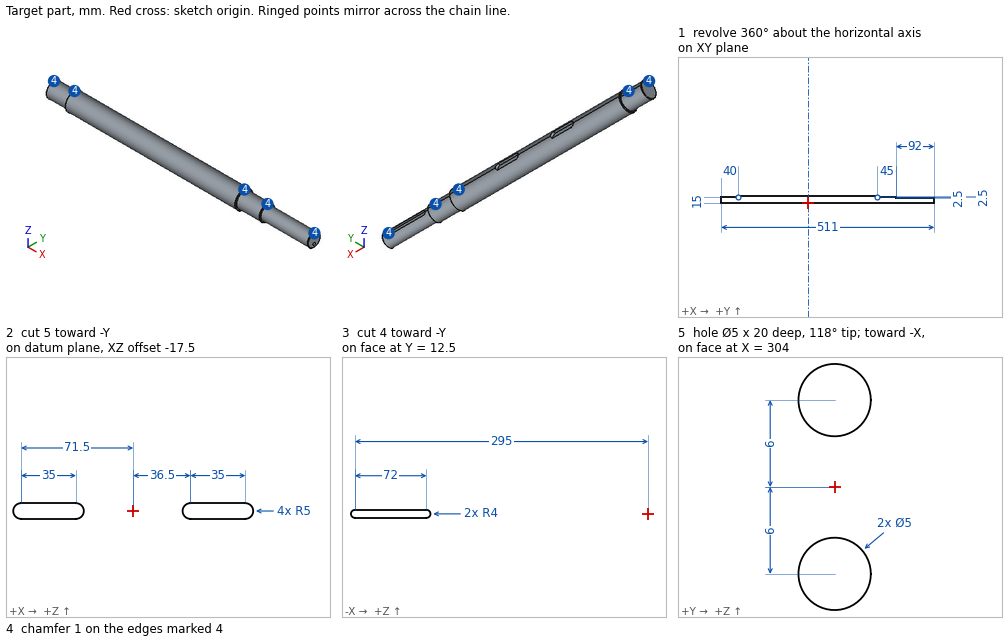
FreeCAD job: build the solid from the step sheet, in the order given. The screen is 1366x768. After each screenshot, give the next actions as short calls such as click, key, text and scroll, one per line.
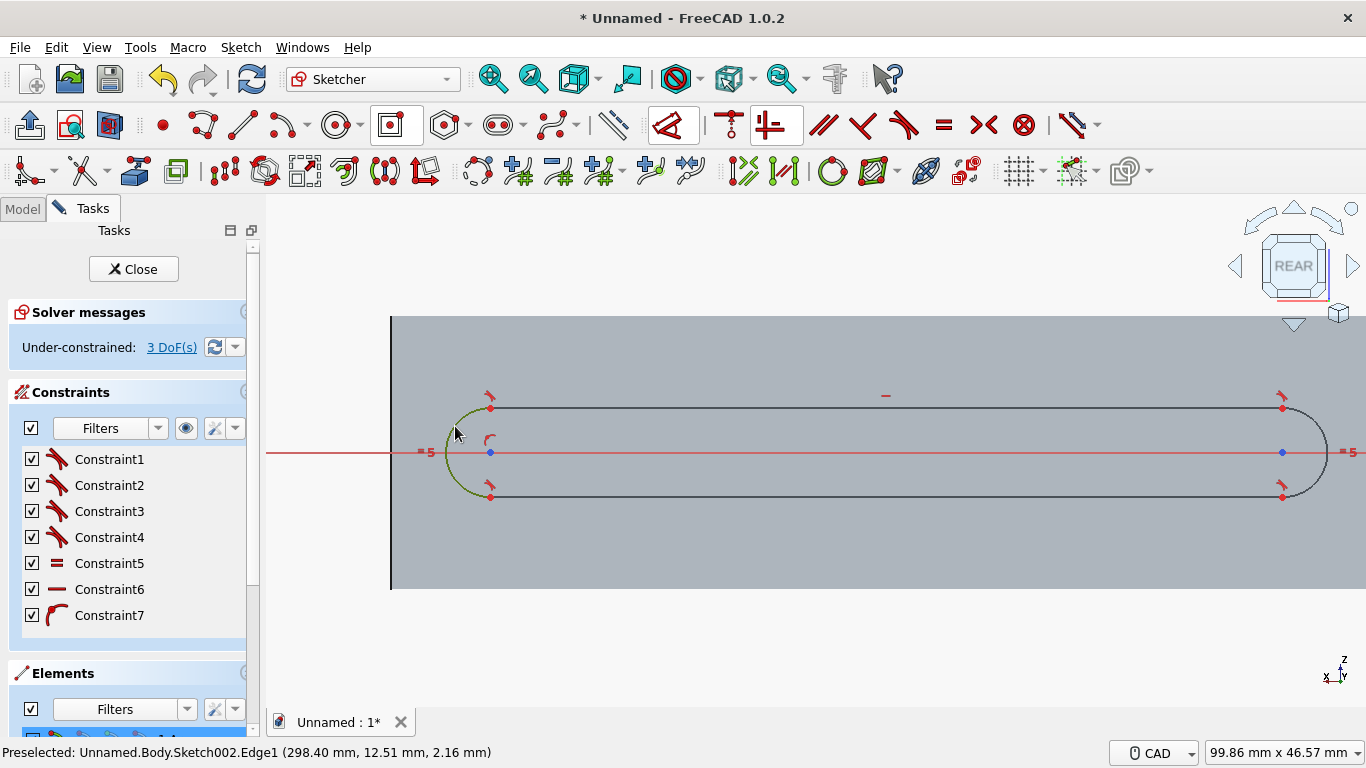
key(k)
key(r)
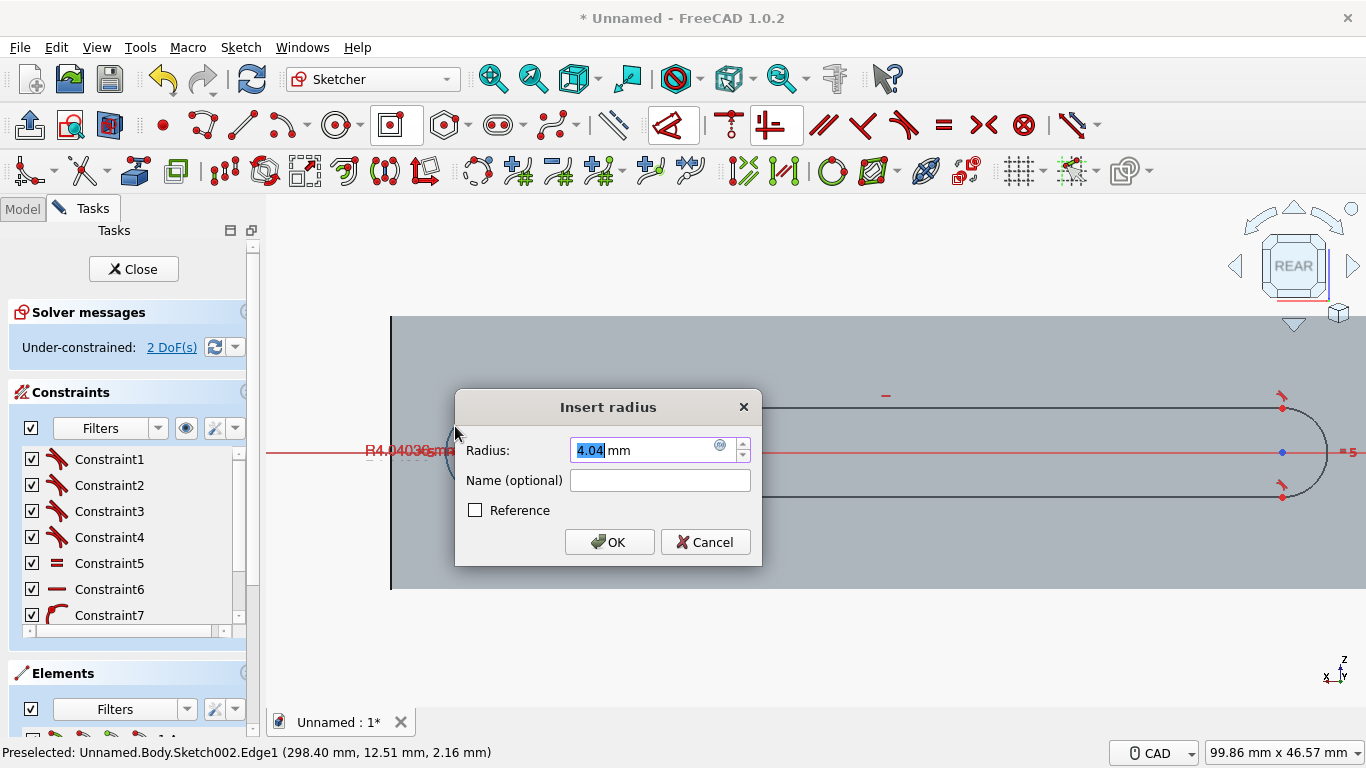
text(4)
key(Return)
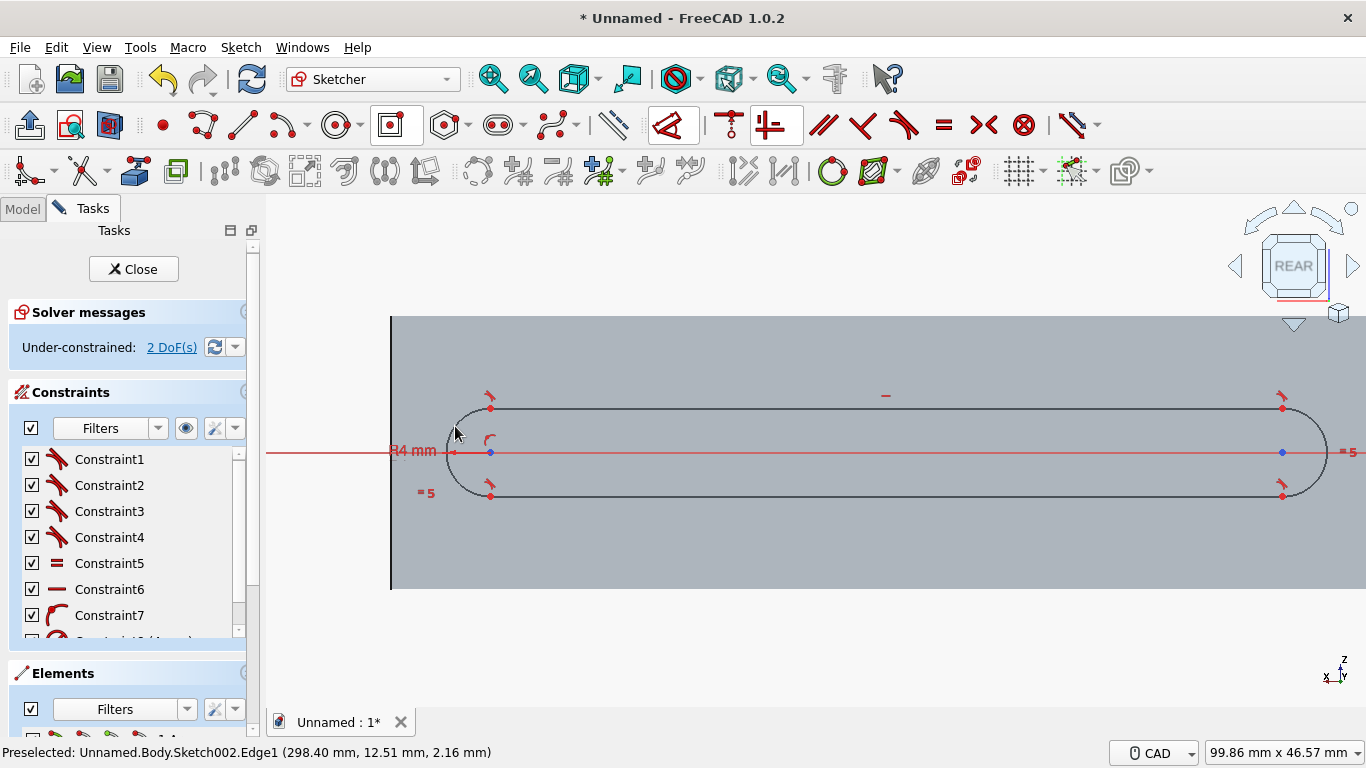
click(728, 409)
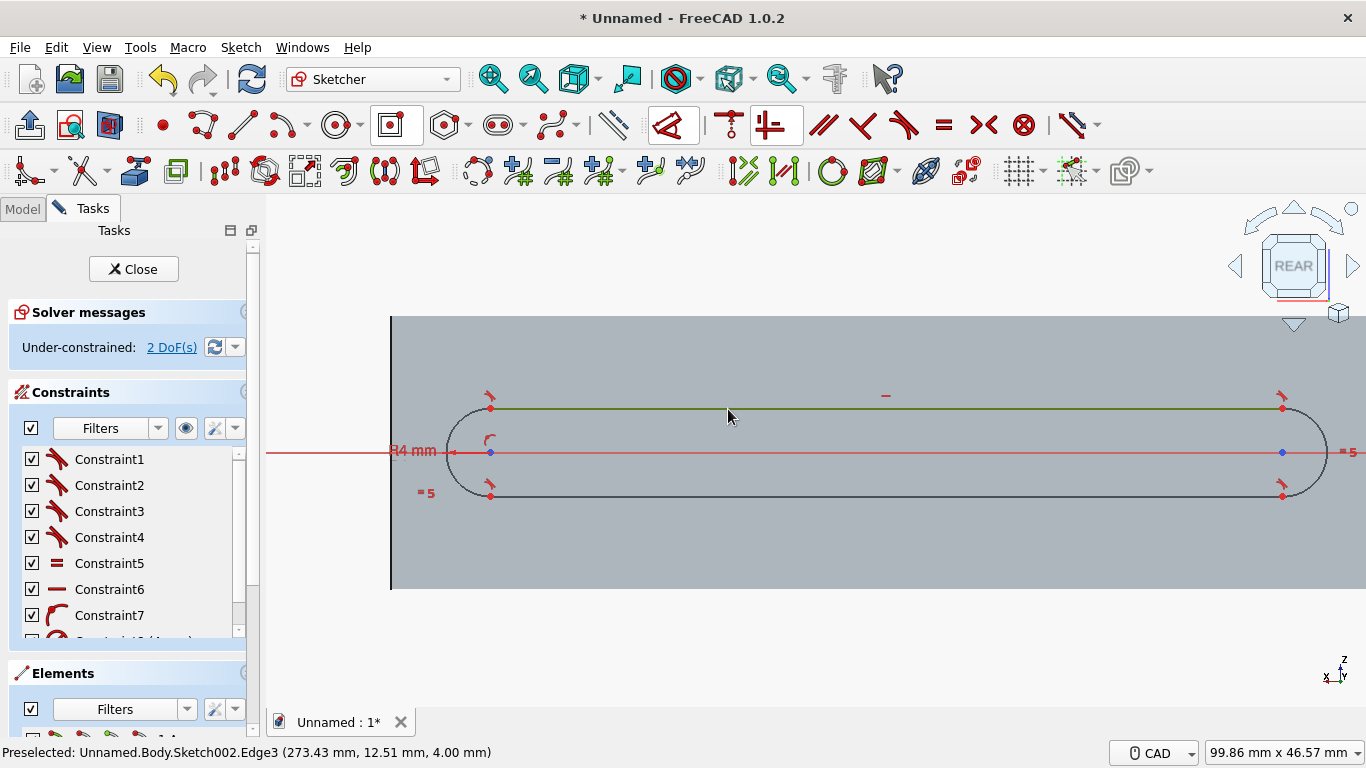
key(l)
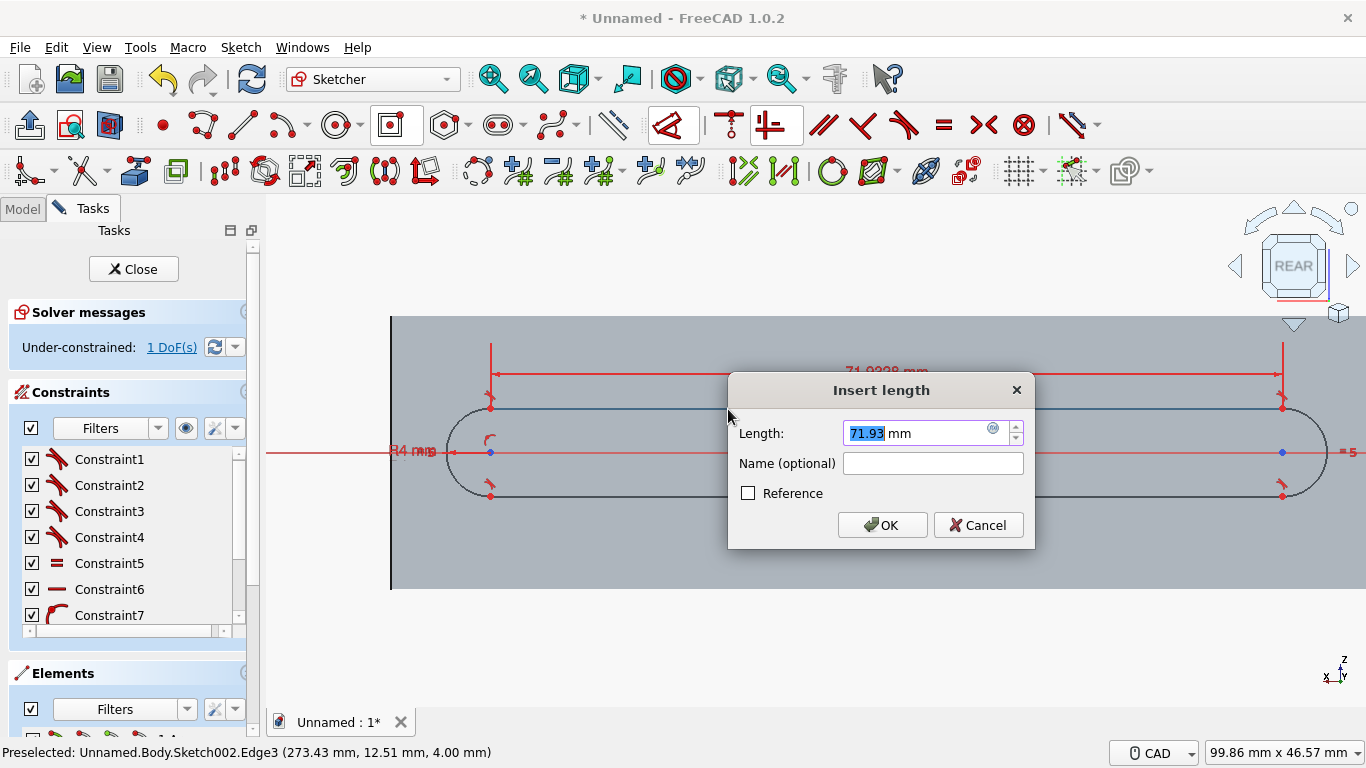
text(72)
key(Return)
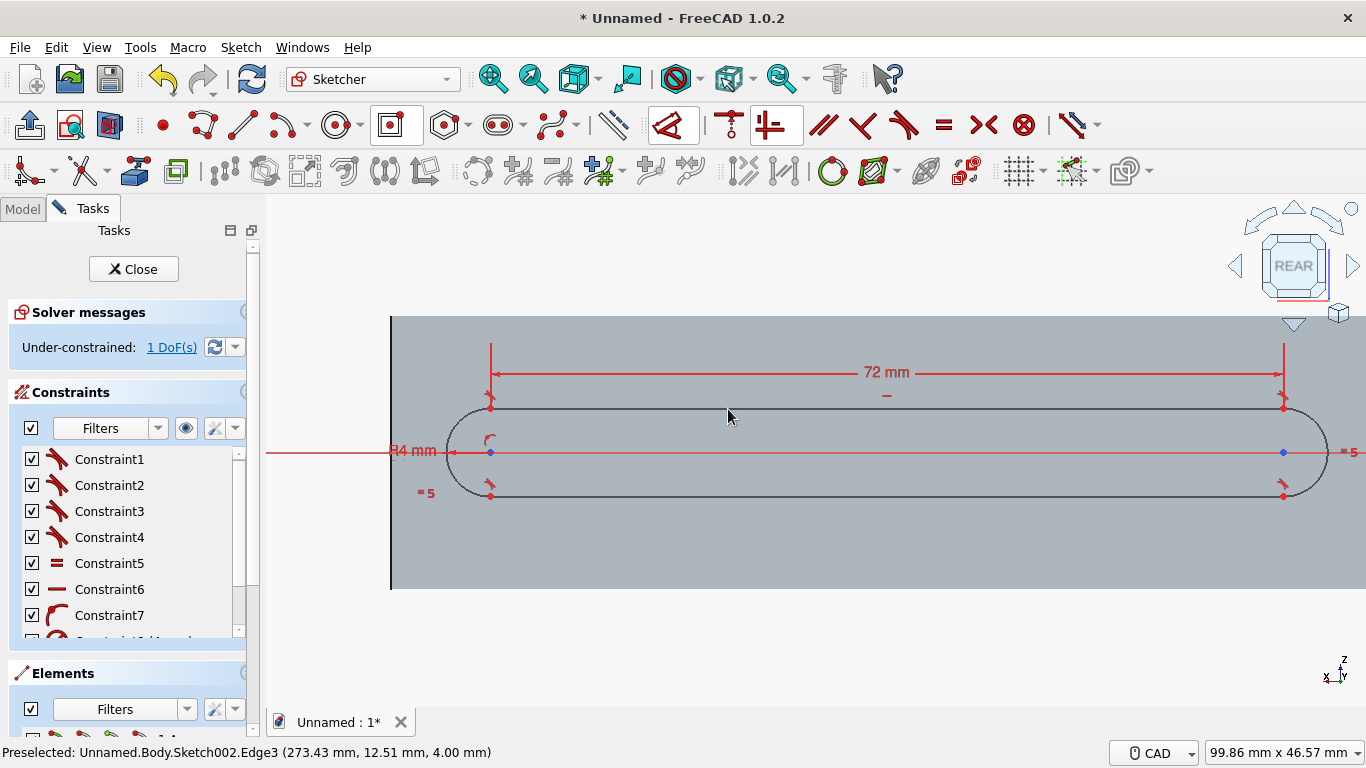
click(491, 409)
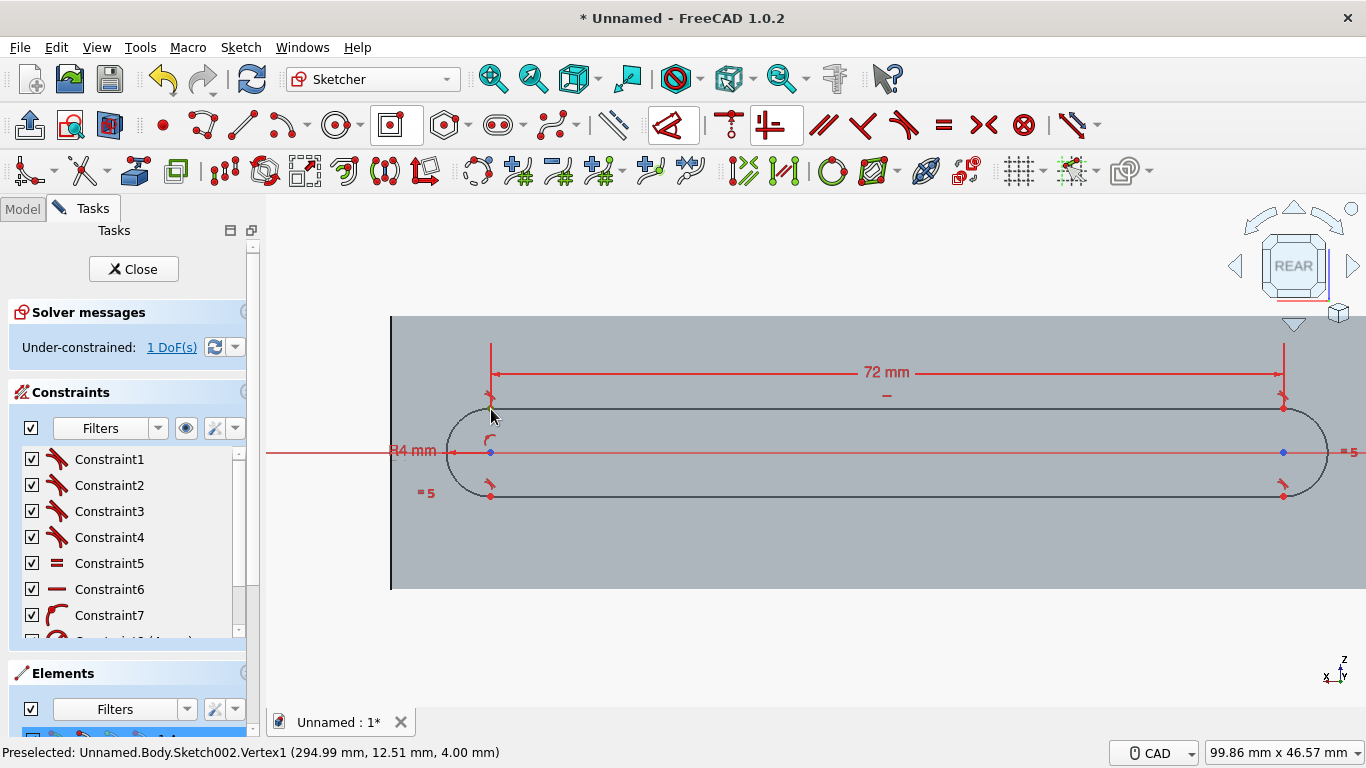
key(l)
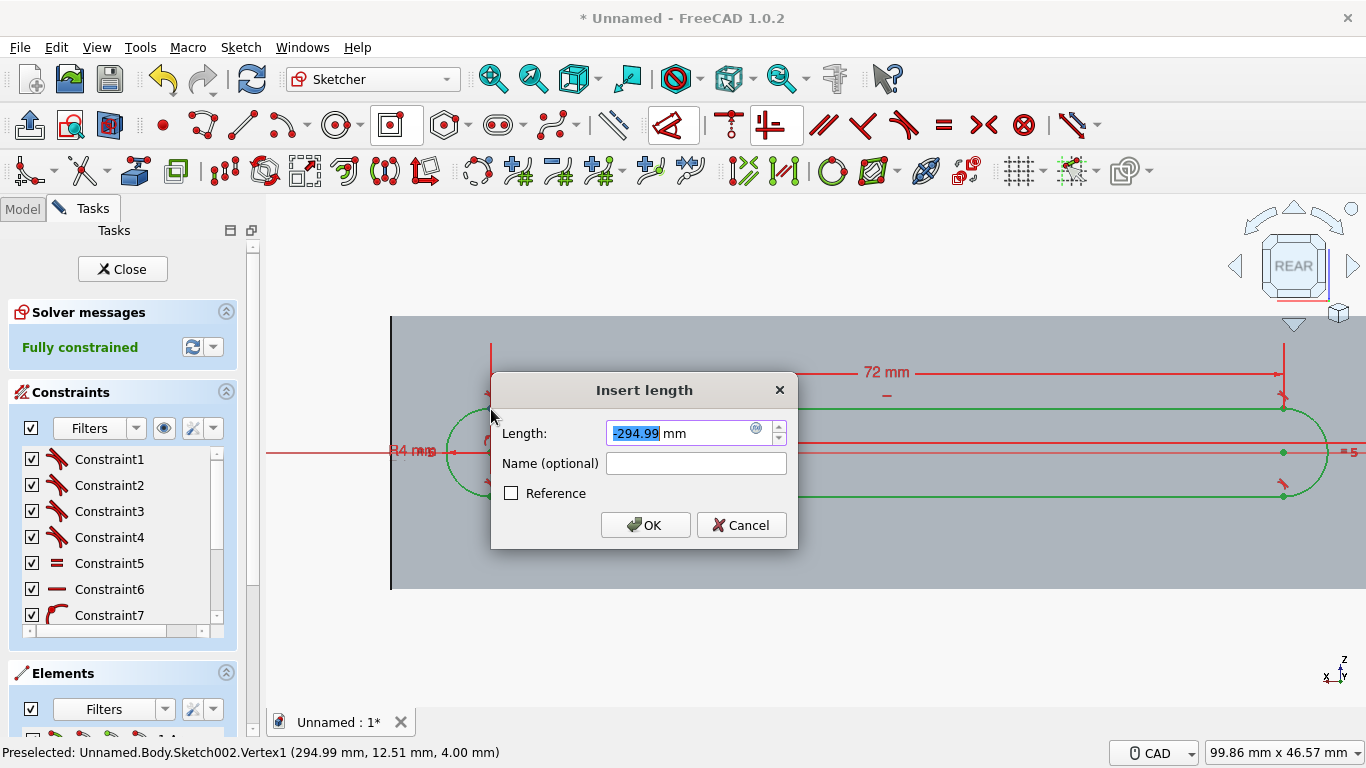
text(-295)
key(Return)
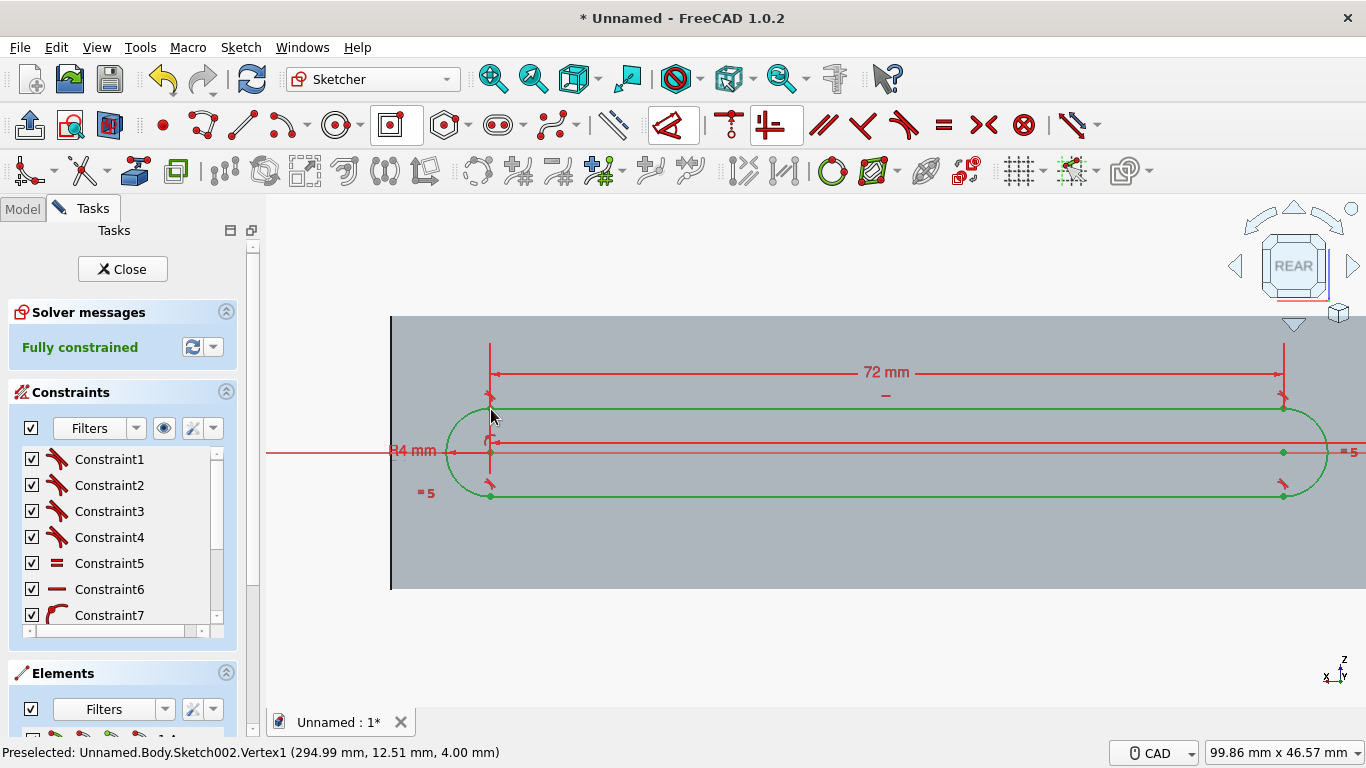
click(123, 269)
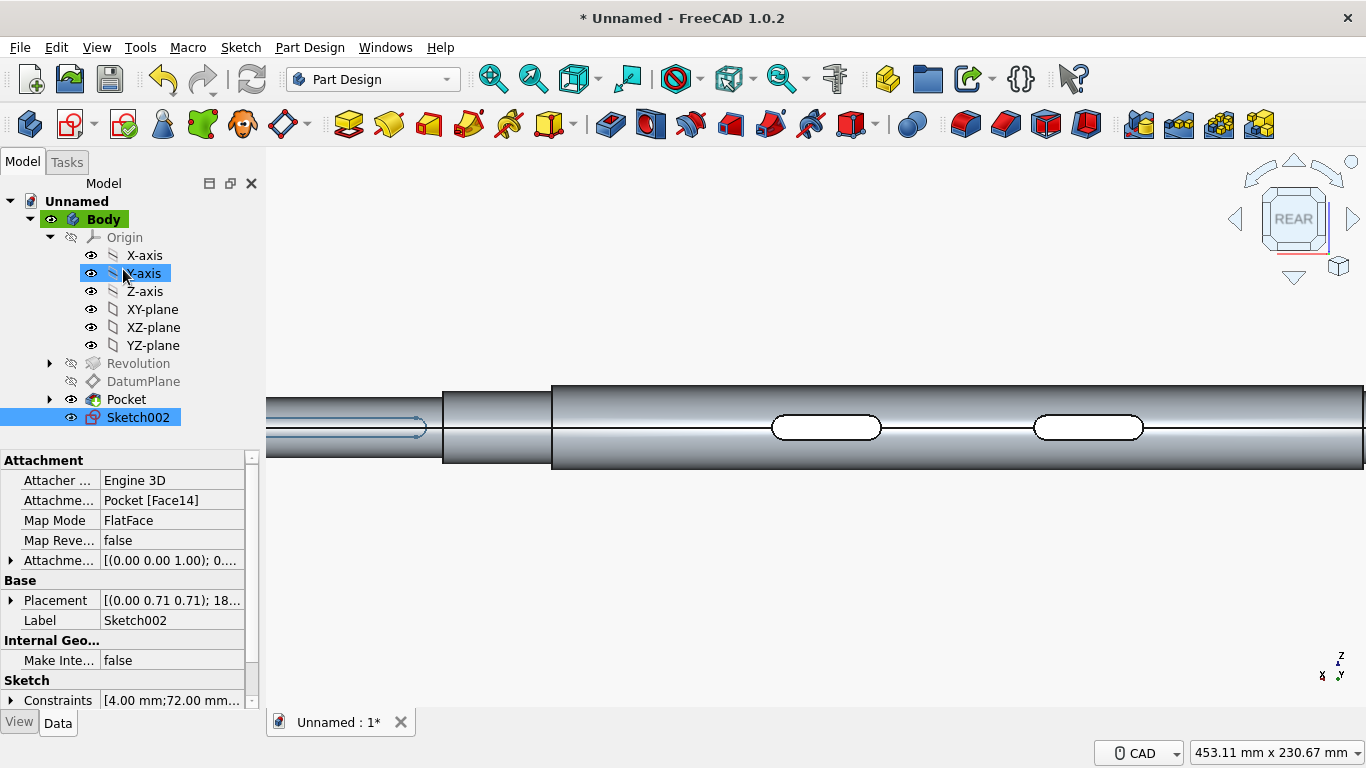
click(612, 124)